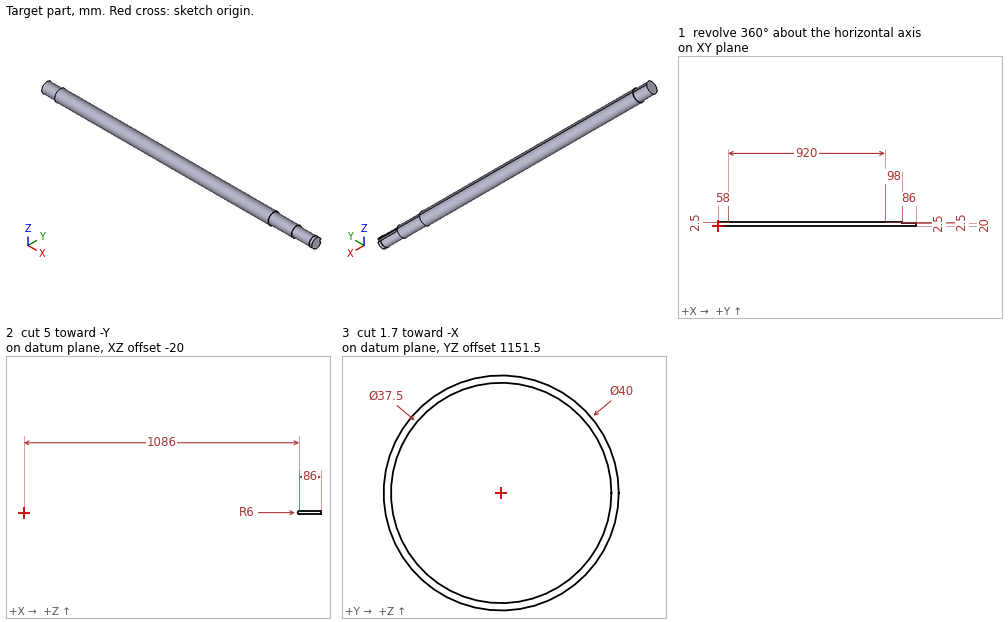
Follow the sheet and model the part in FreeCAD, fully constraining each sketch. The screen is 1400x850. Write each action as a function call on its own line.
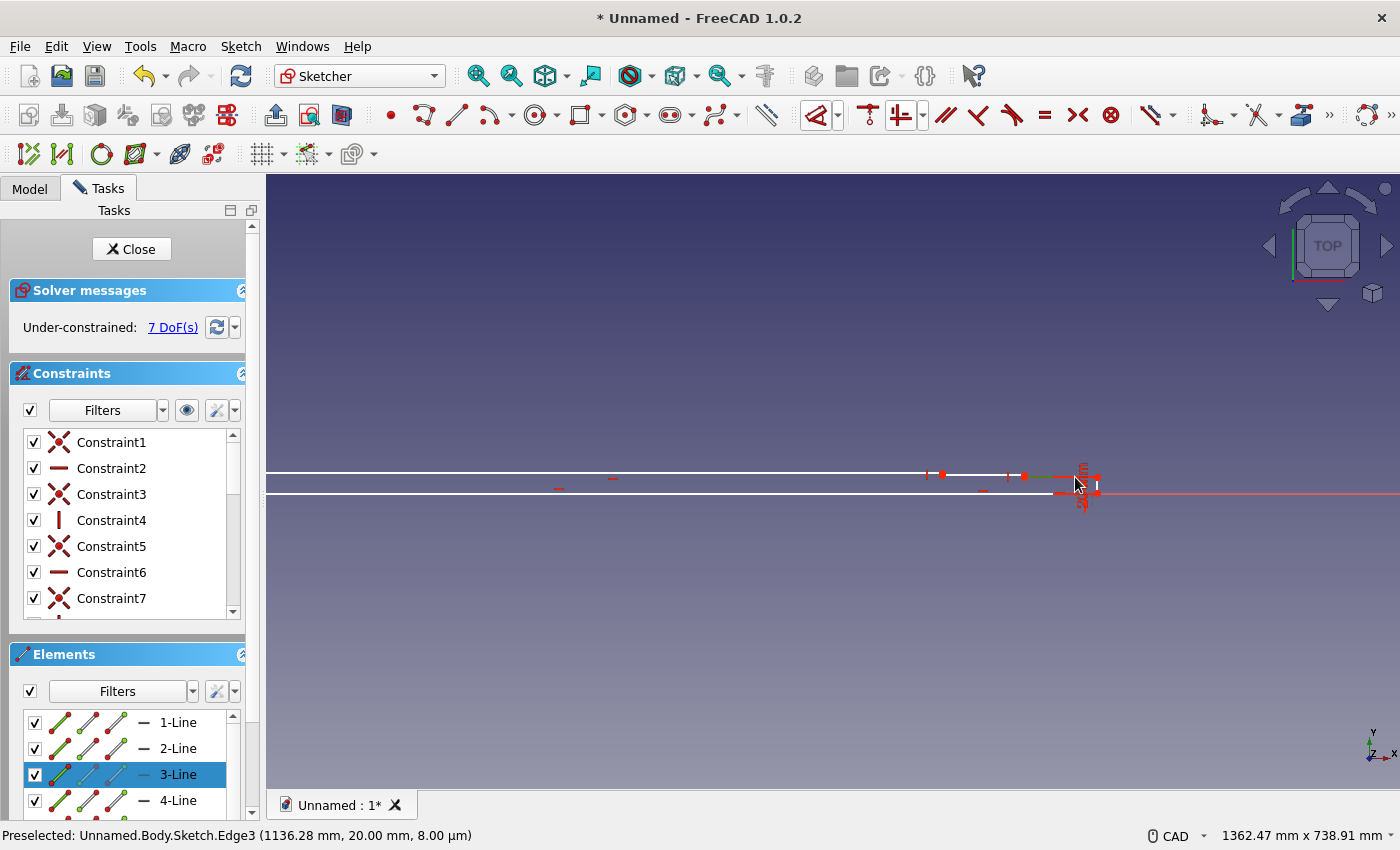
key(l)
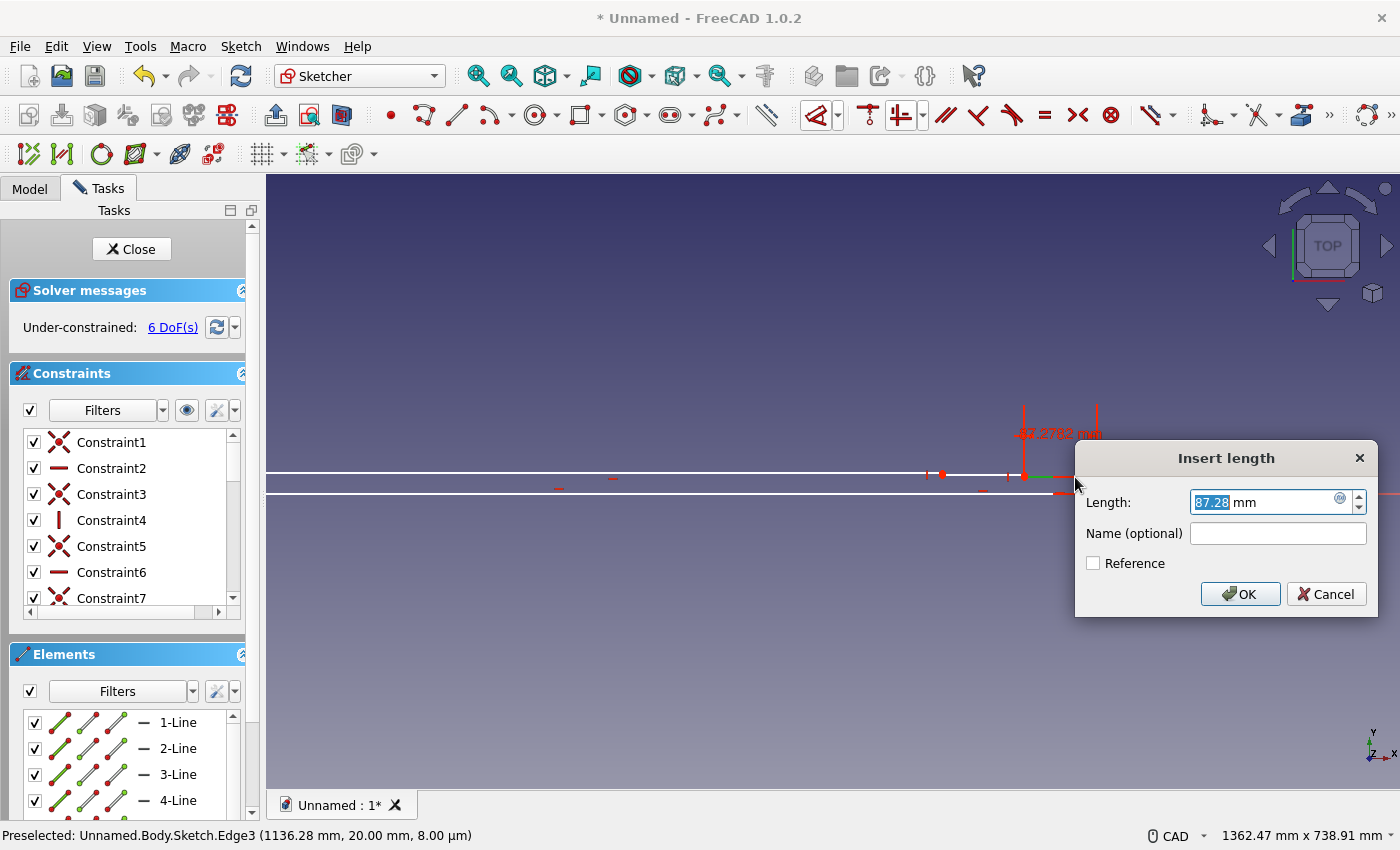
text(86)
key(Return)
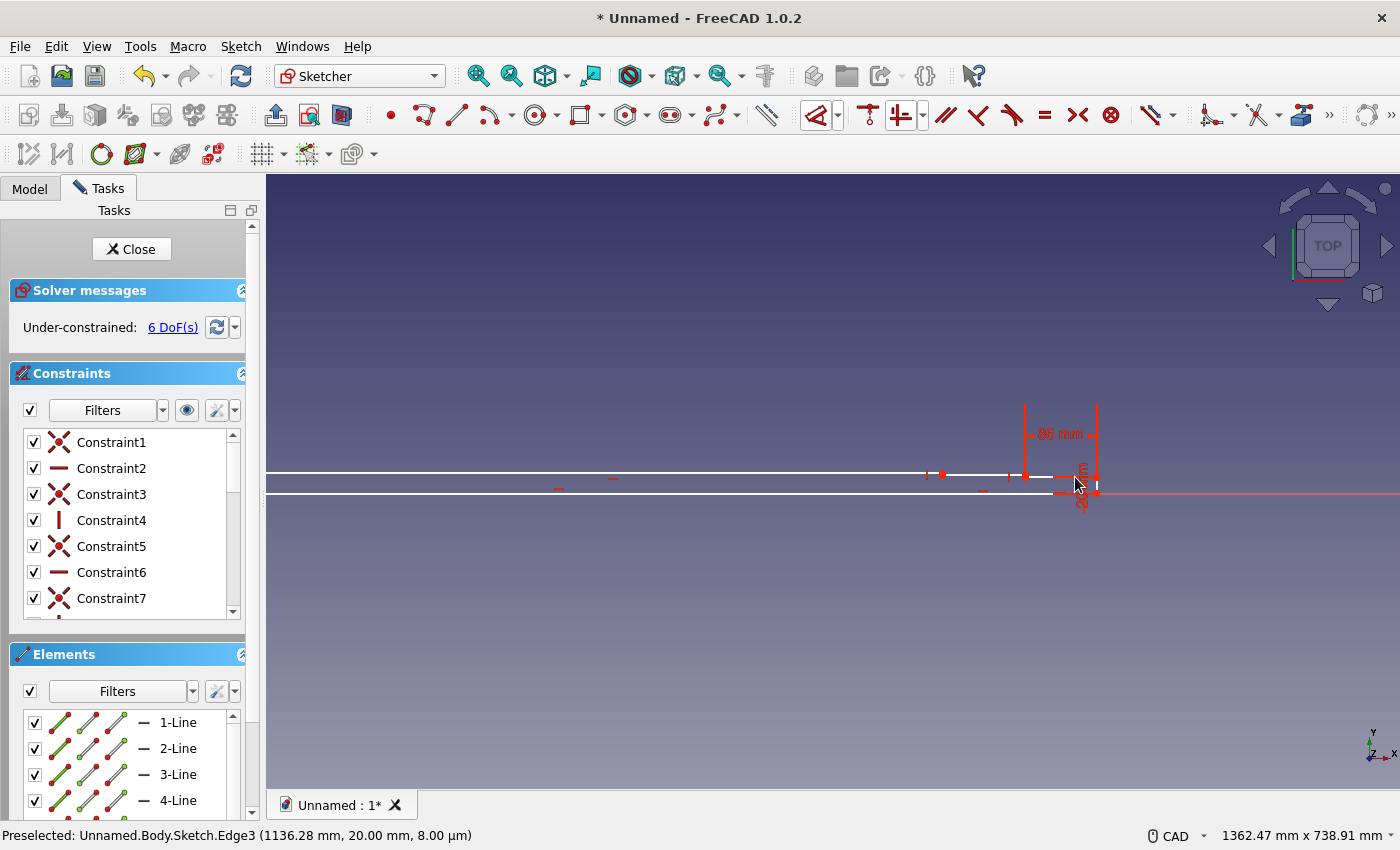
click(1000, 475)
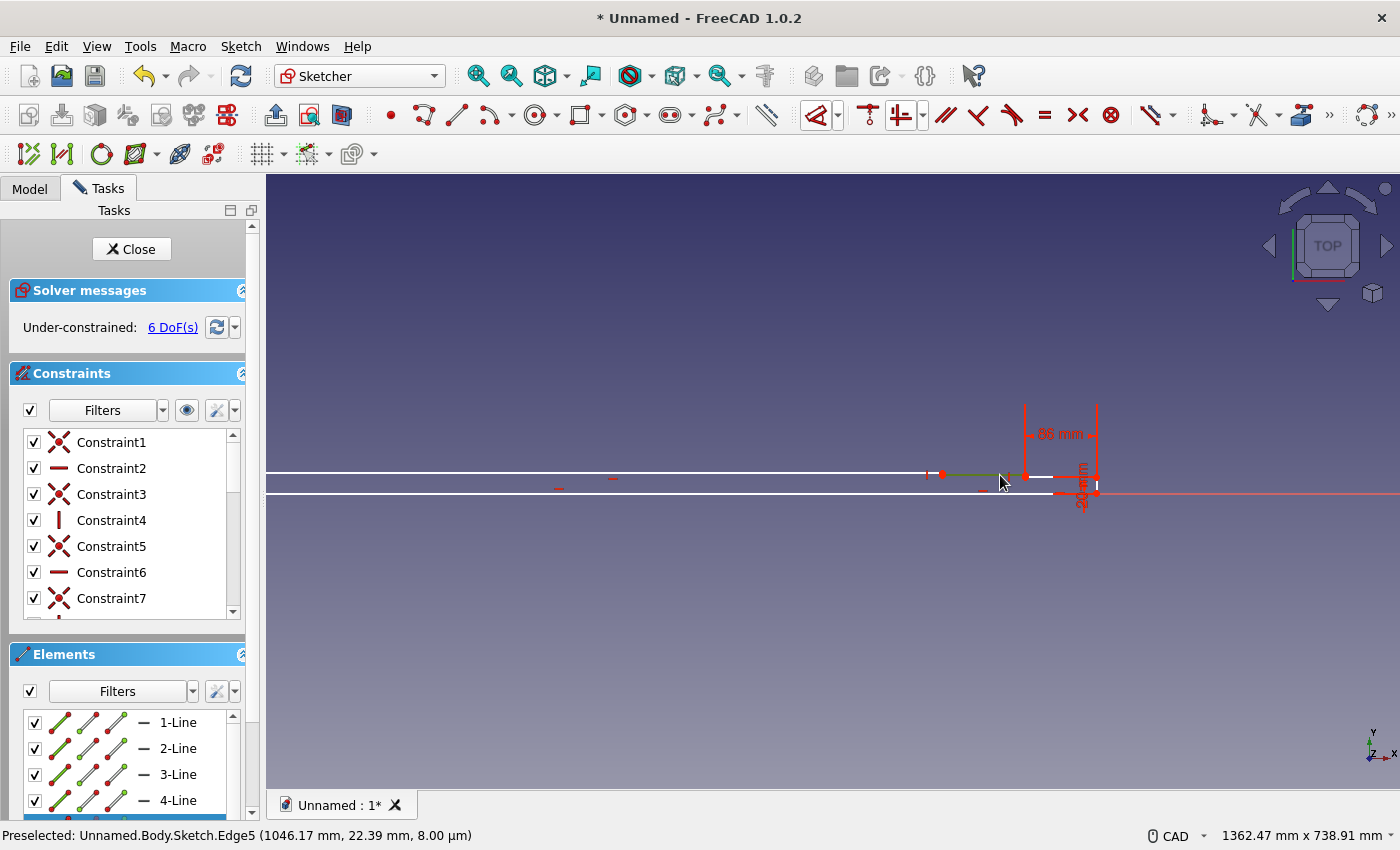
click(838, 116)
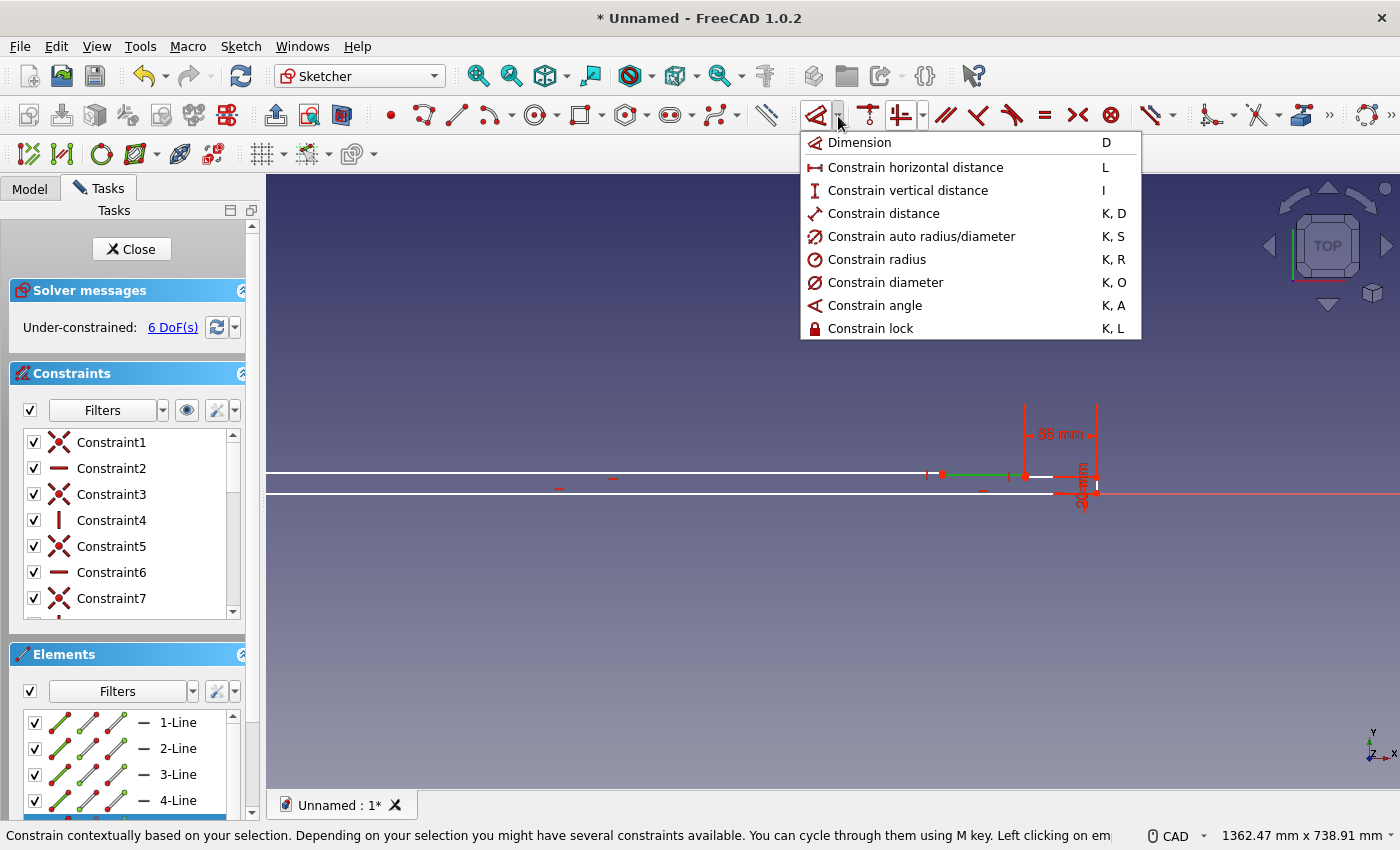
click(971, 168)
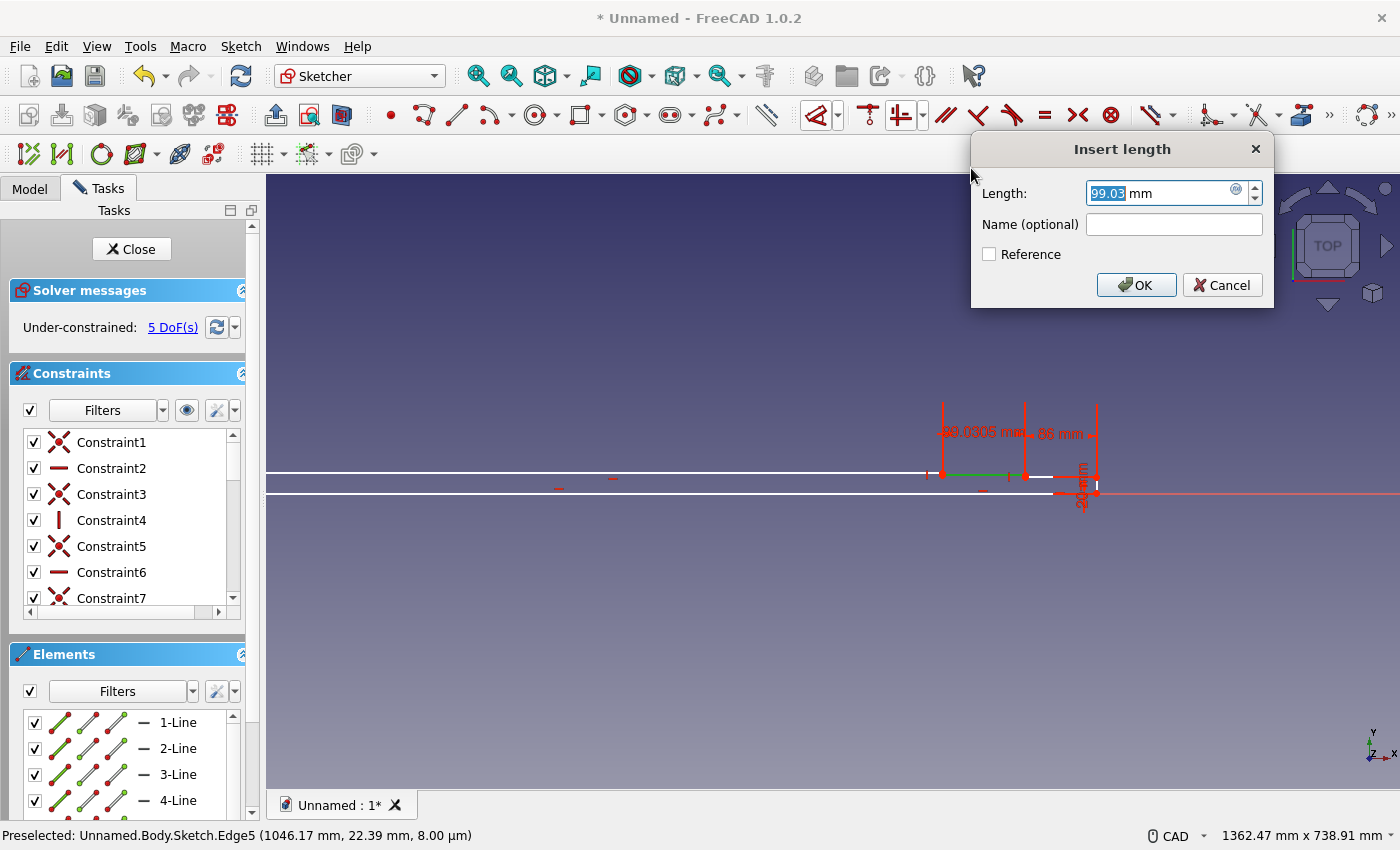
text(98)
key(Return)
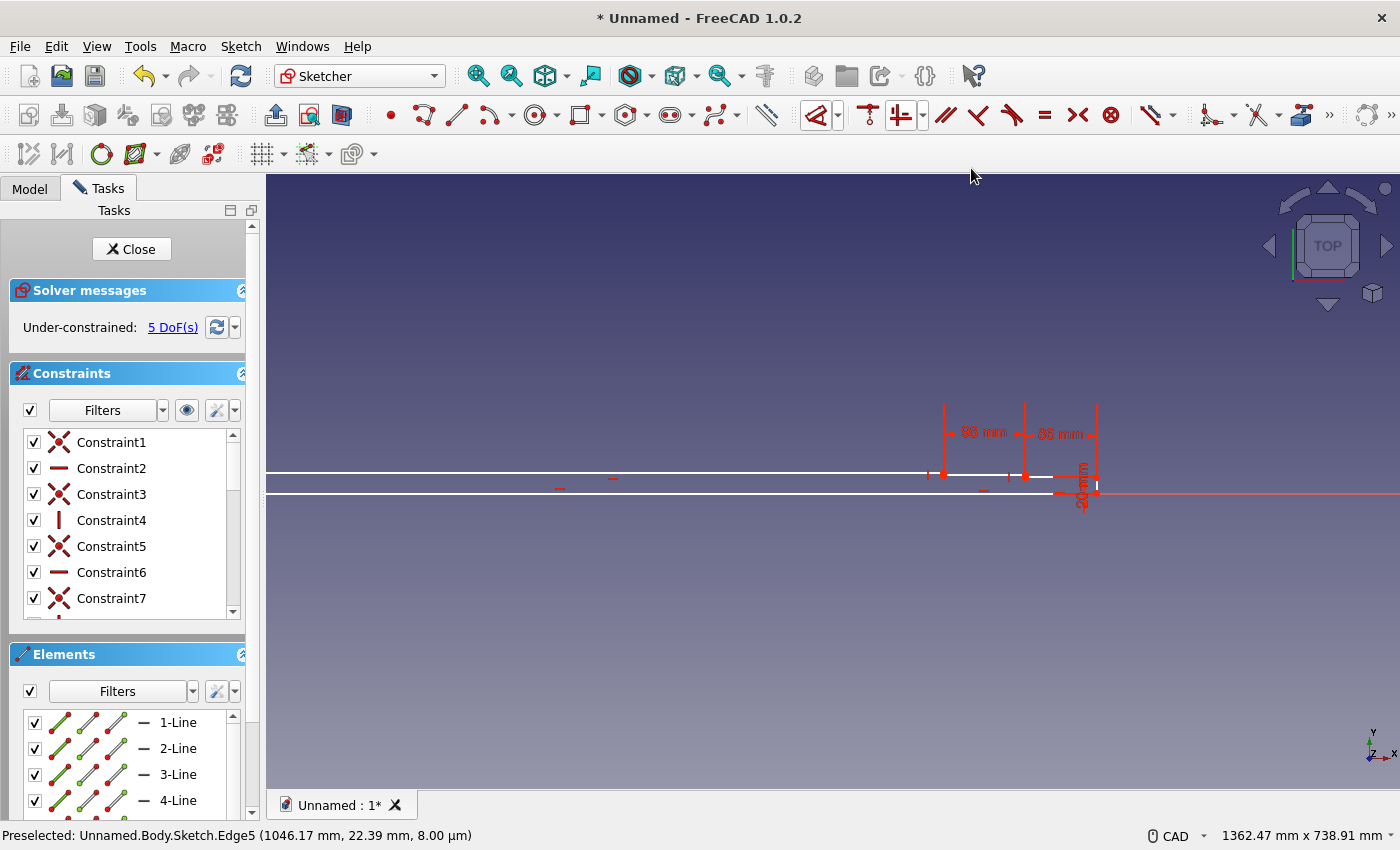
scroll(1073, 478, down, 2)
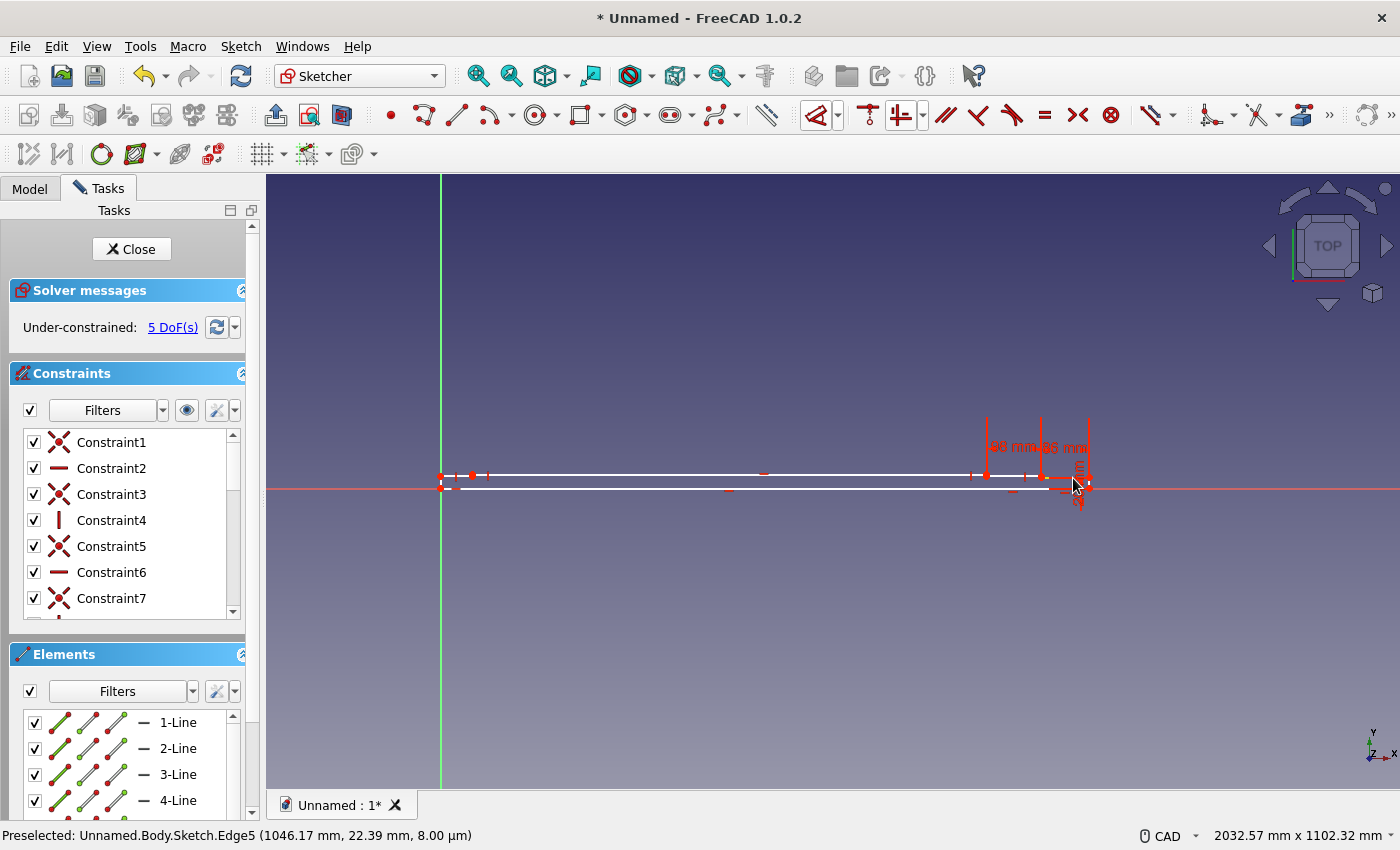
scroll(463, 476, up, 2)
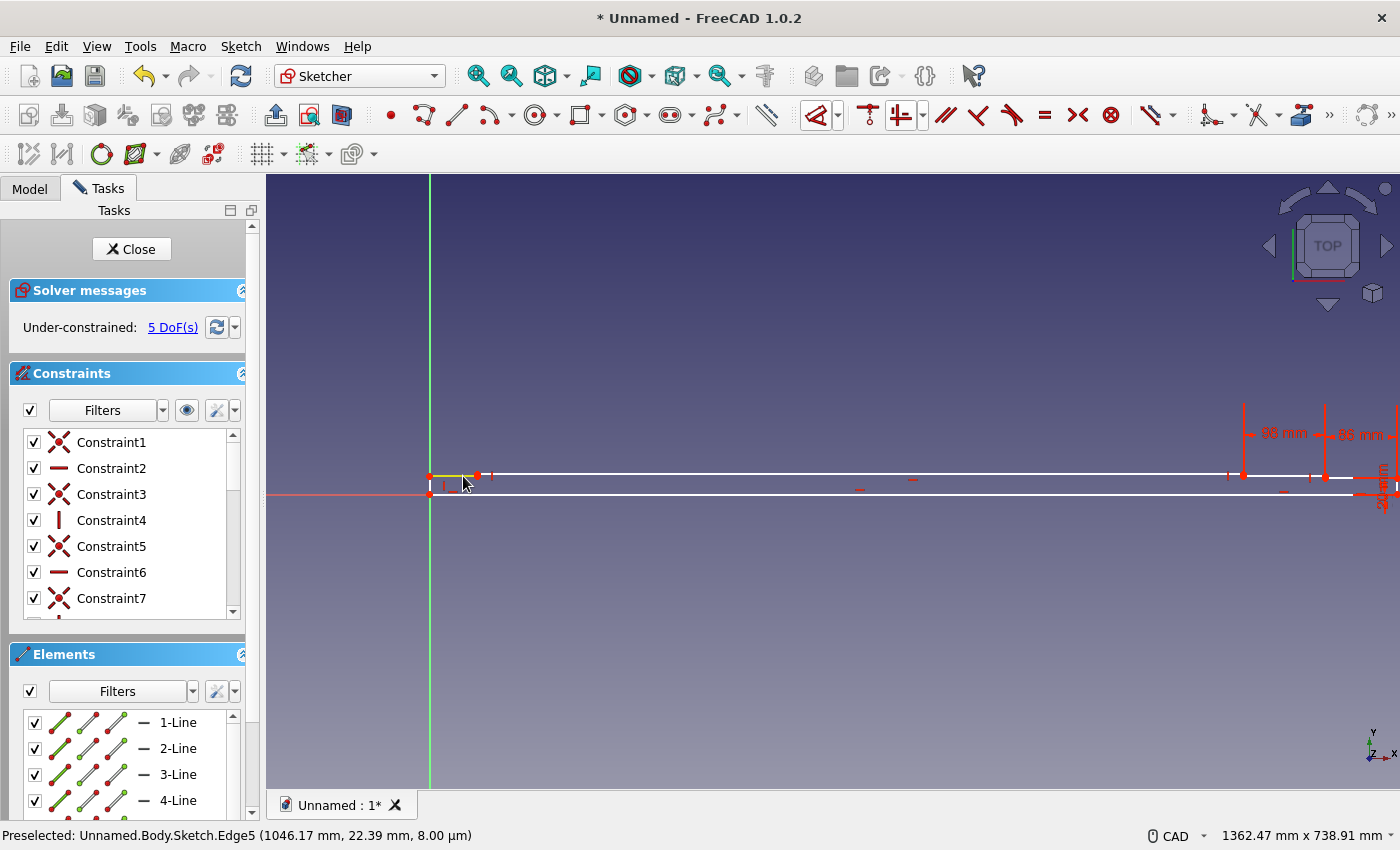
click(463, 476)